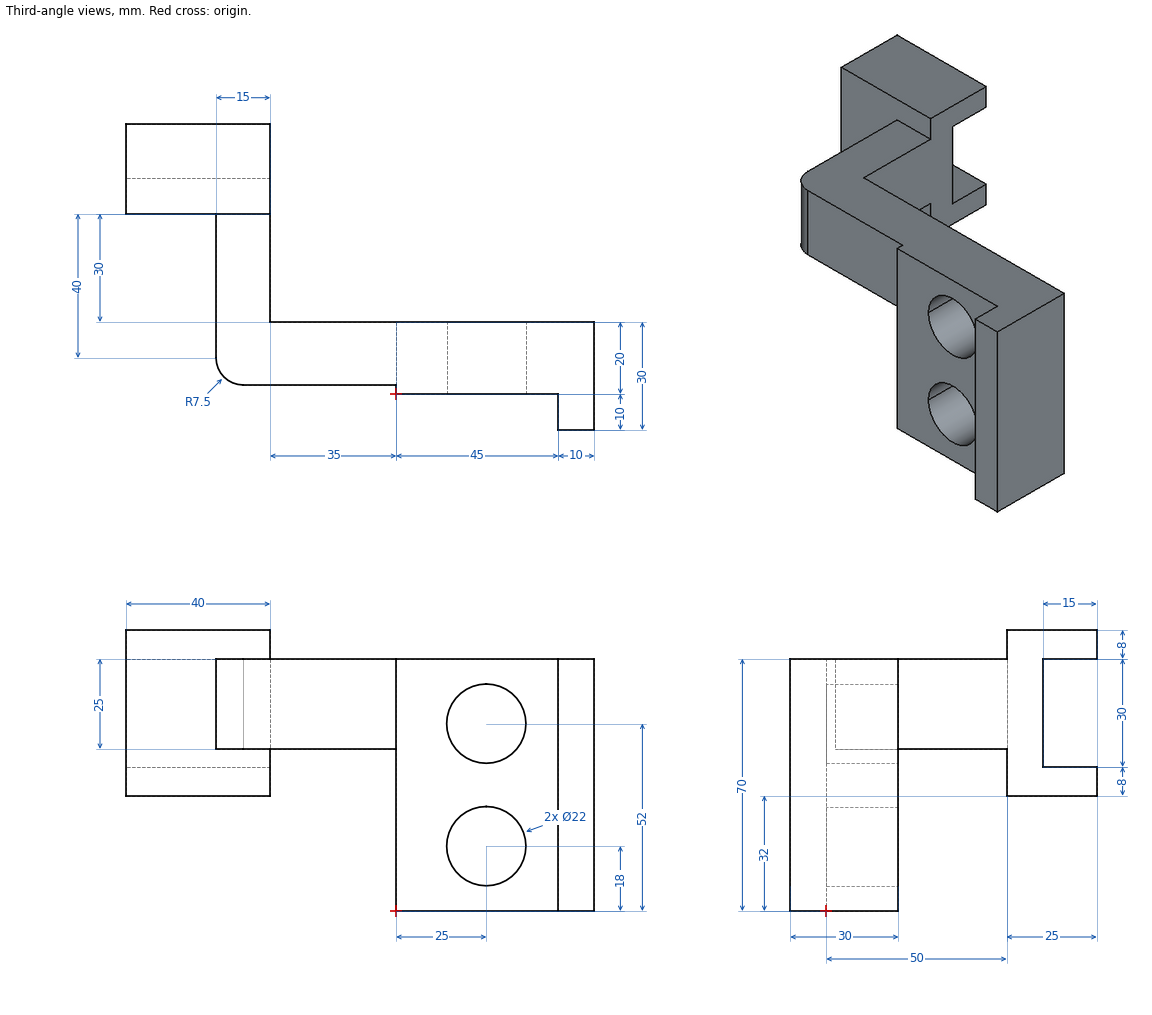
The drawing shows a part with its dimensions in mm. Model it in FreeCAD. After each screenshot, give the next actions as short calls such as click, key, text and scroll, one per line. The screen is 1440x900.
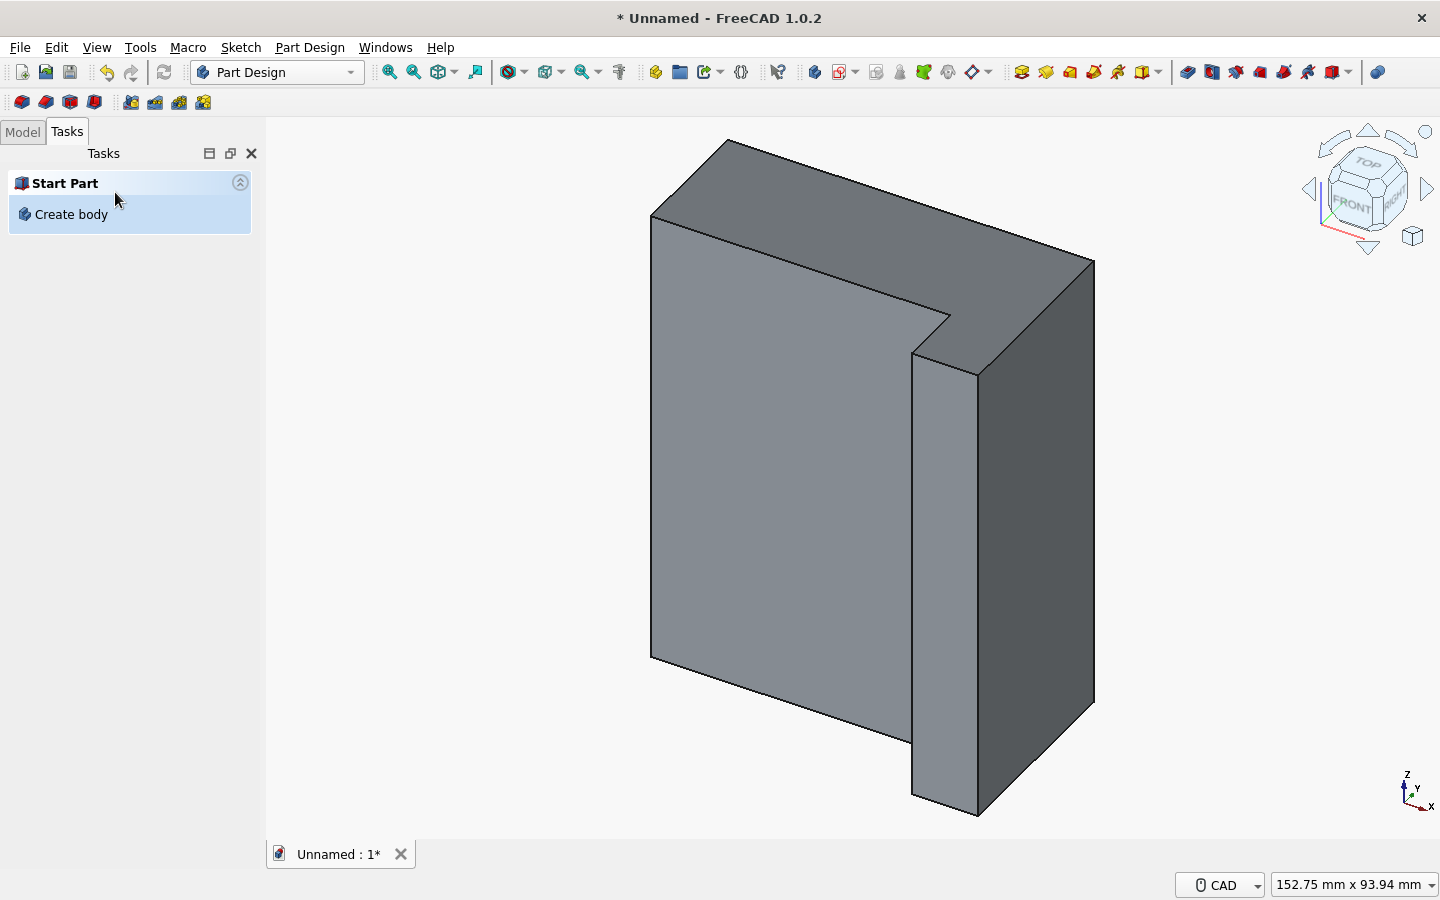
click(974, 275)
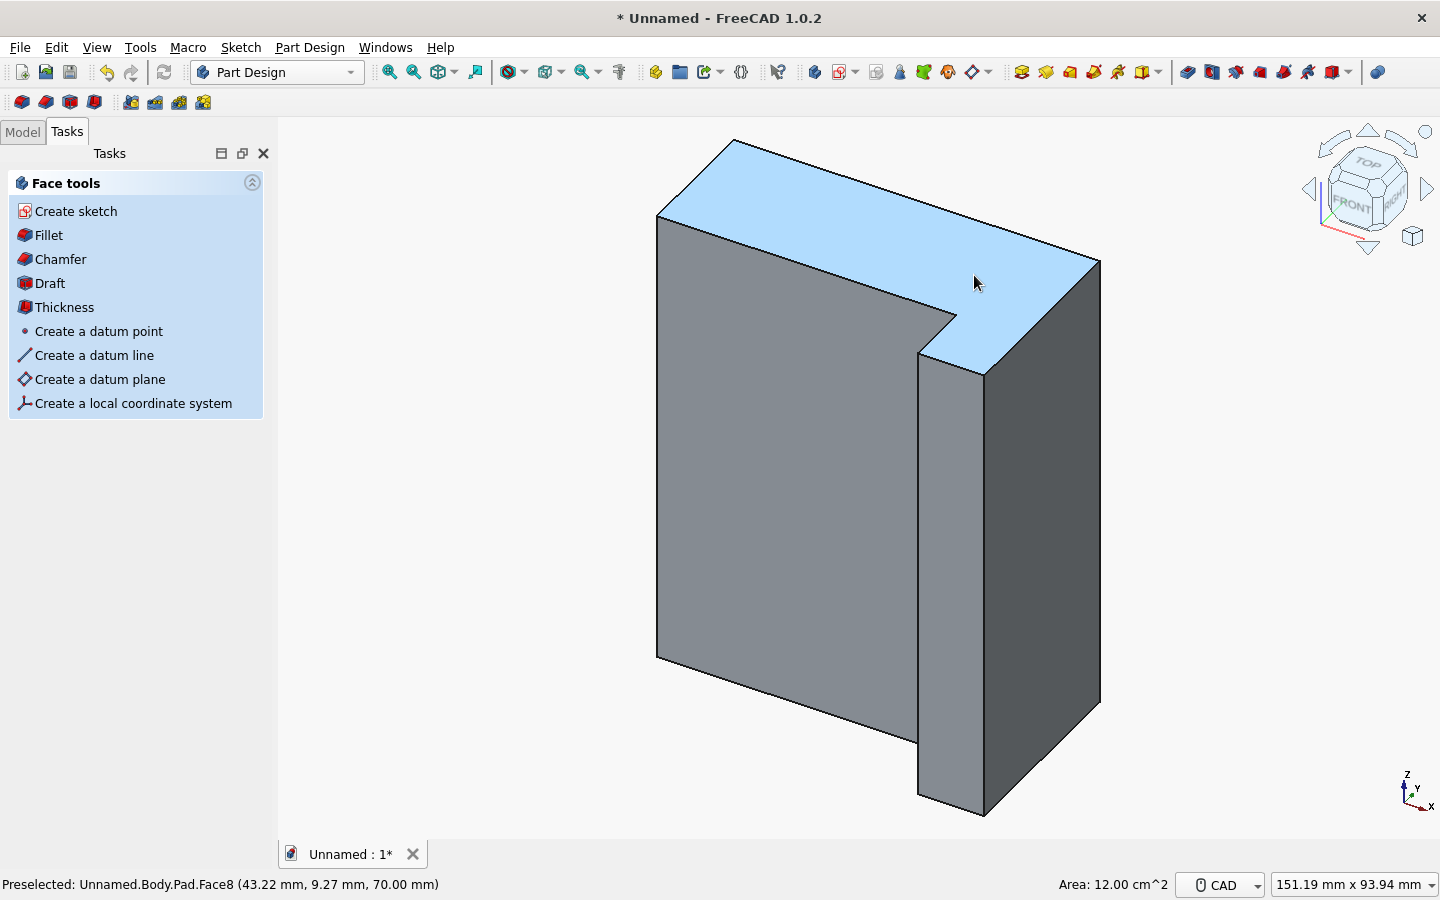
click(840, 72)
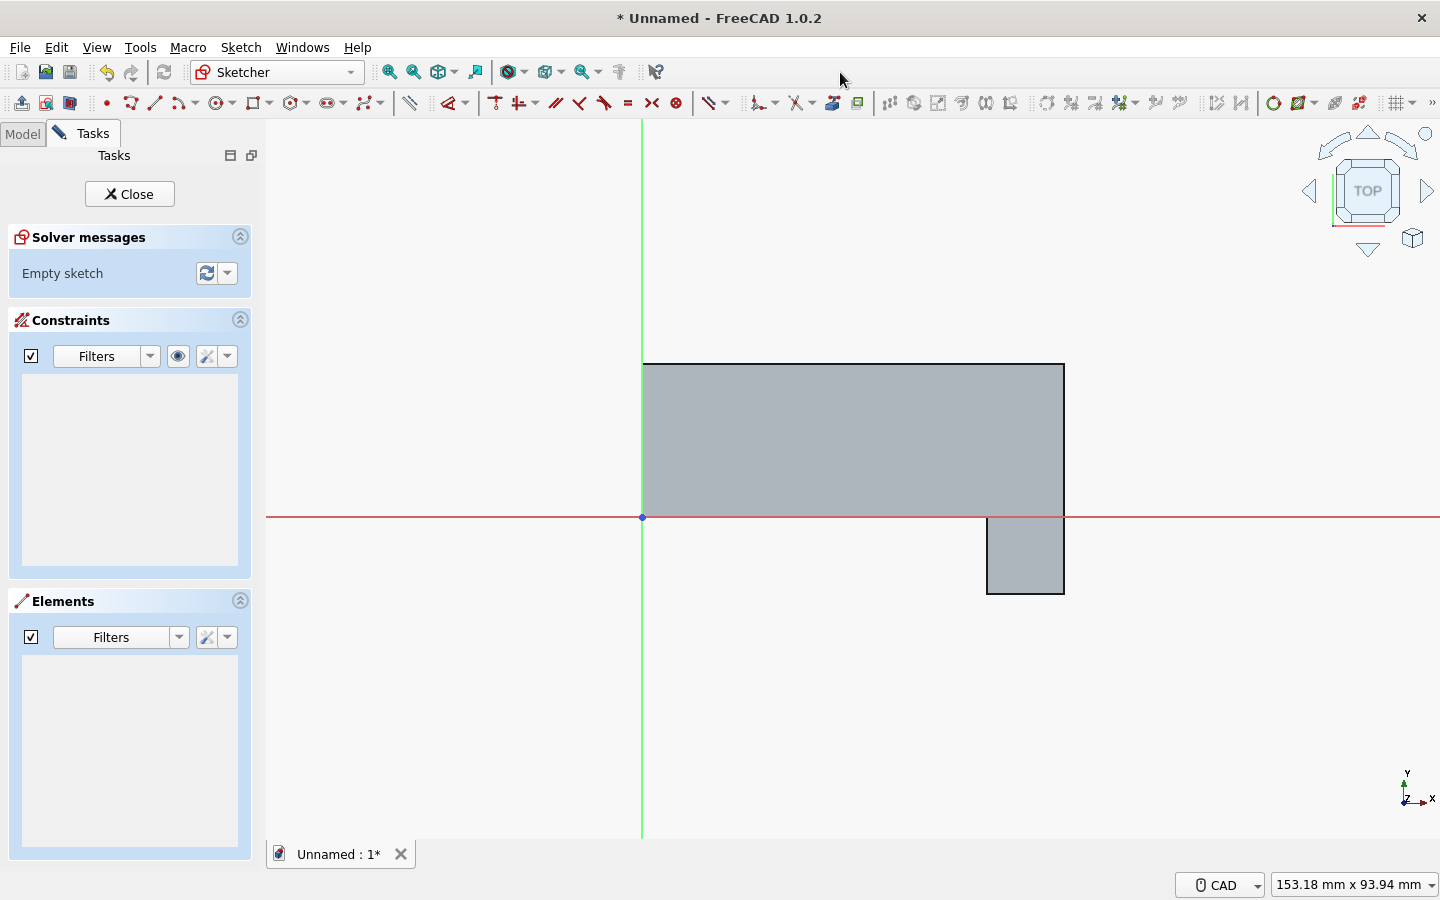
scroll(1275, 811, down, 1)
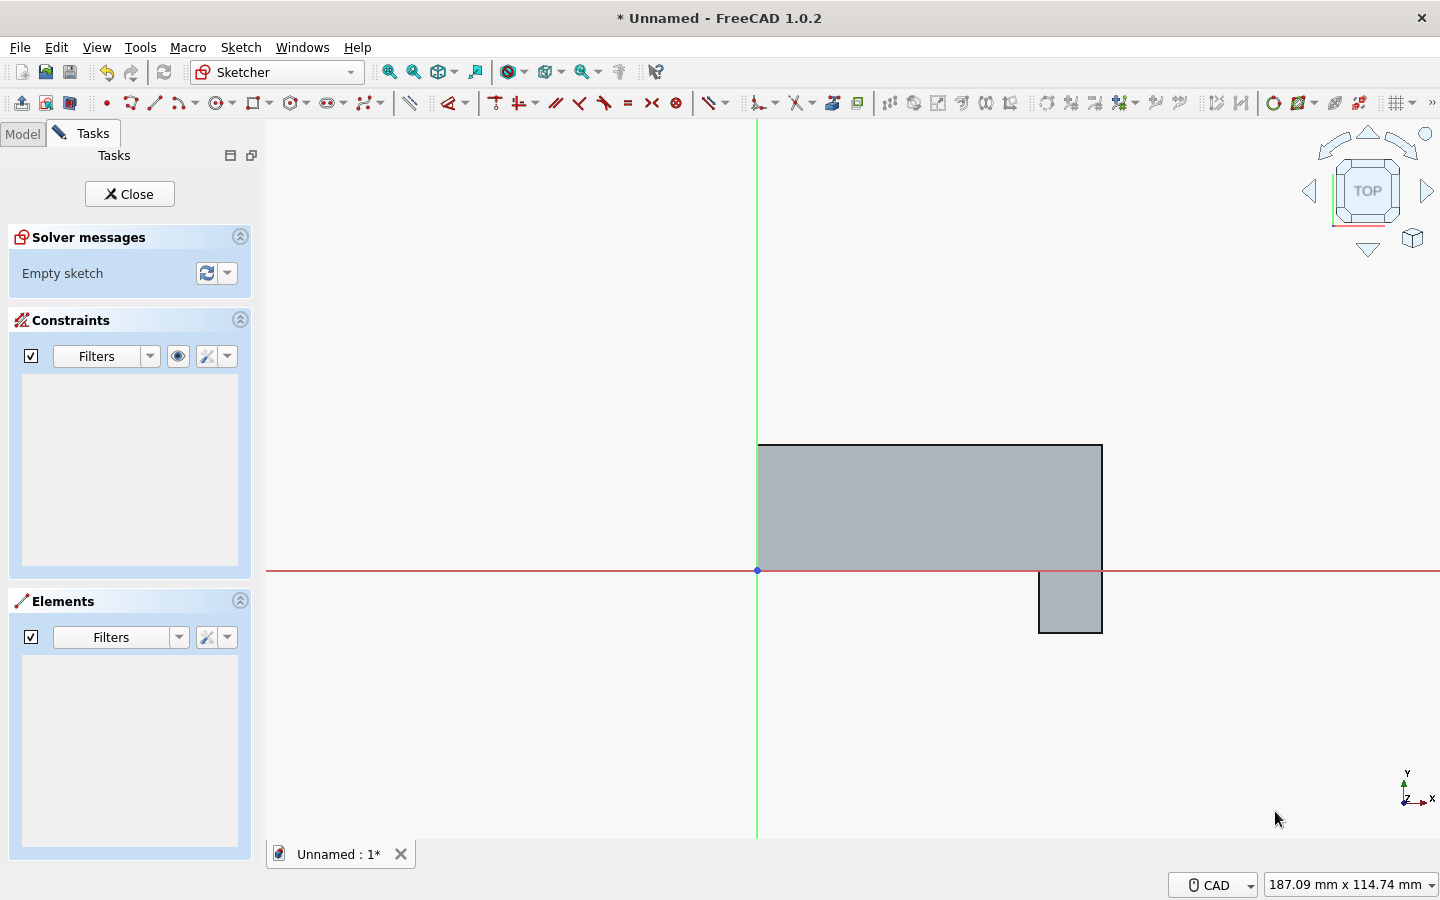
scroll(294, 281, up, 2)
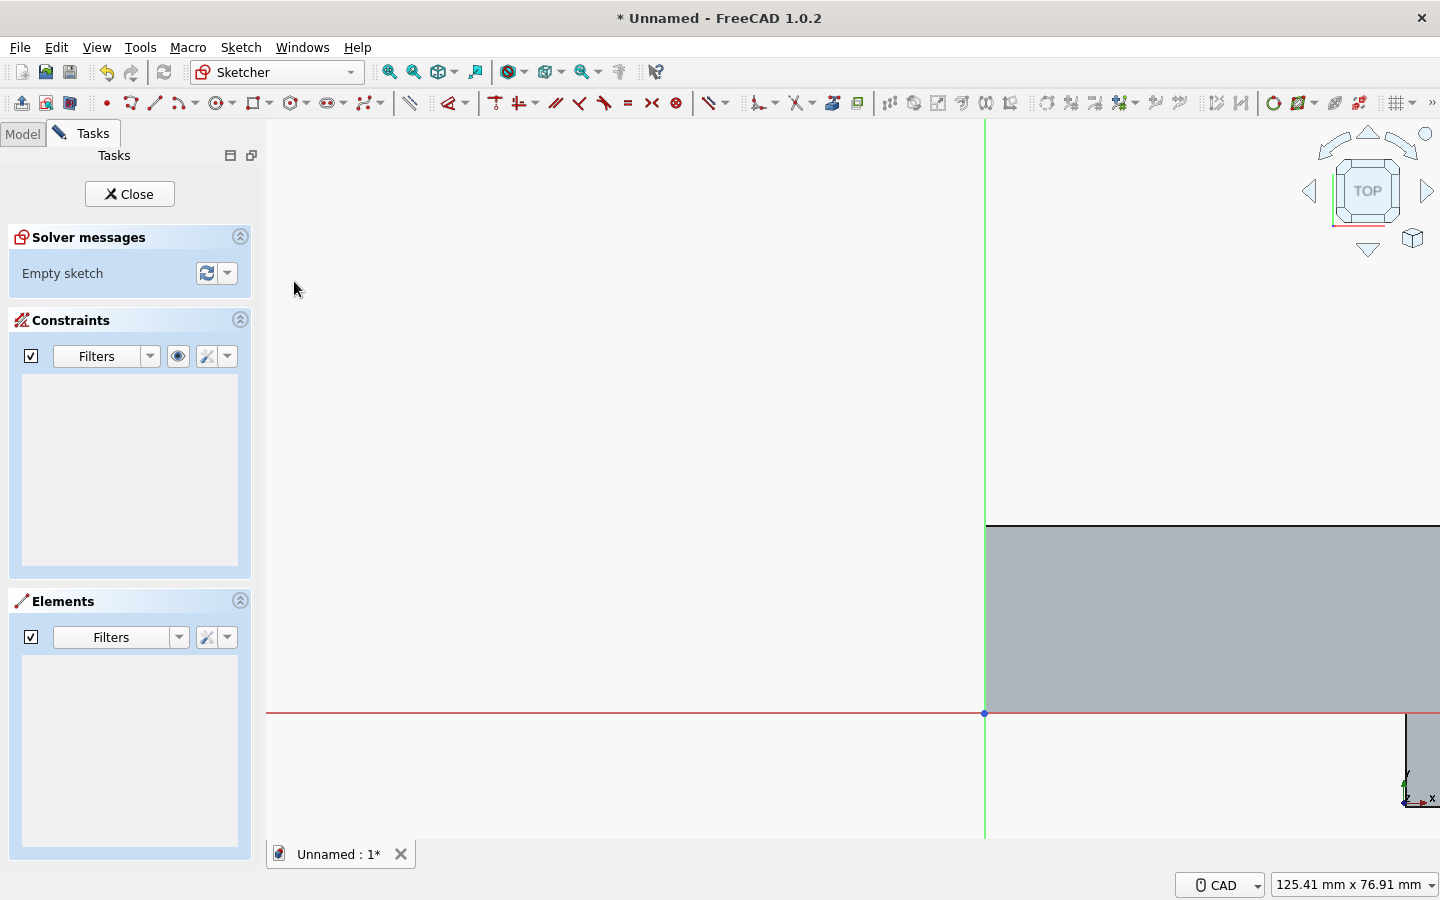
click(132, 104)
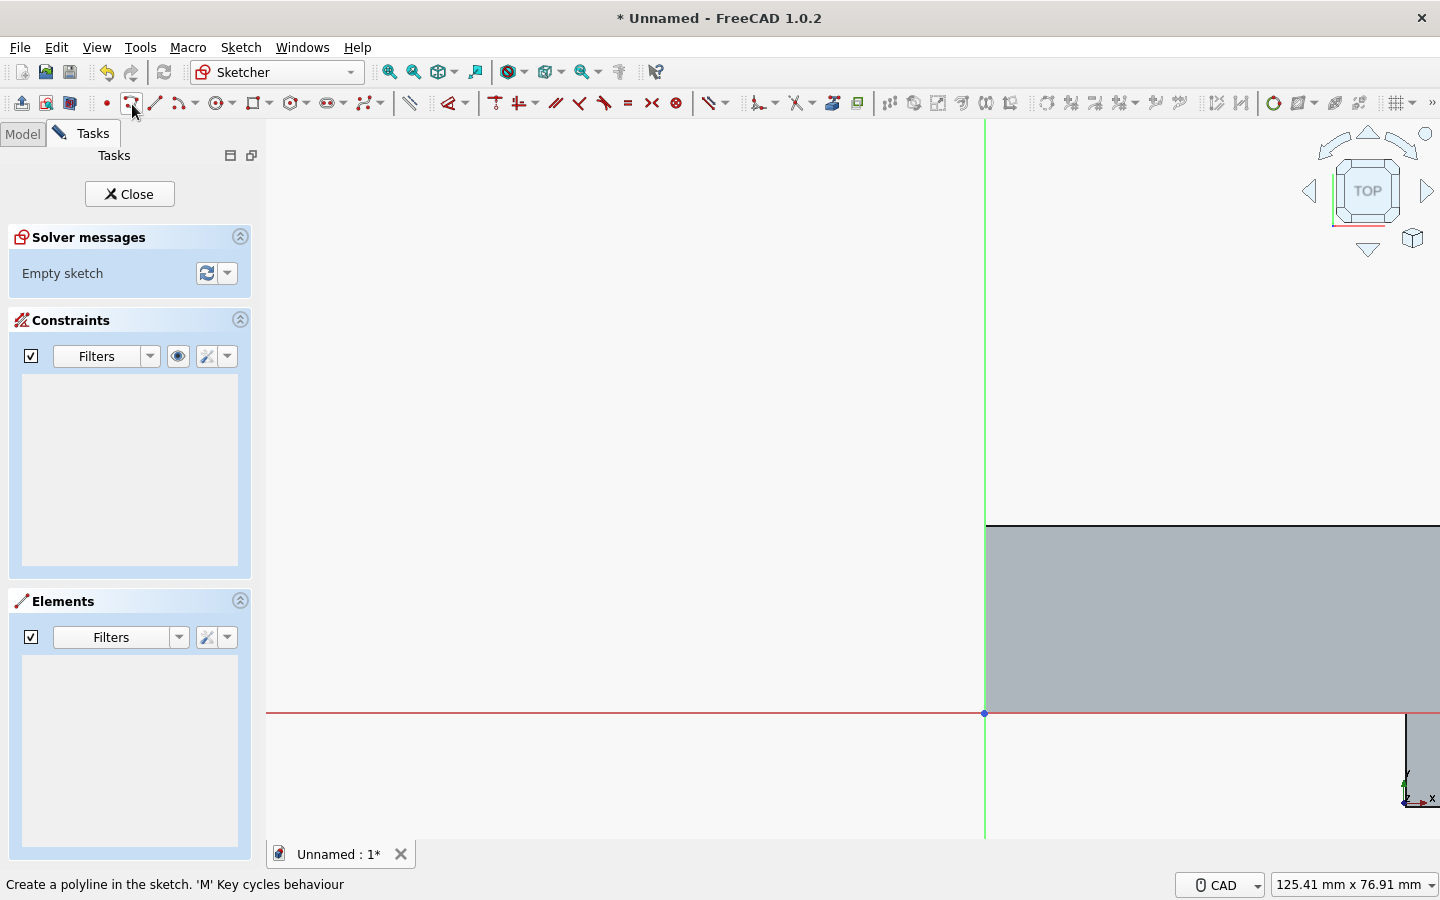
click(587, 690)
click(985, 690)
click(976, 526)
click(657, 526)
click(657, 245)
click(517, 245)
click(517, 620)
right_click(517, 620)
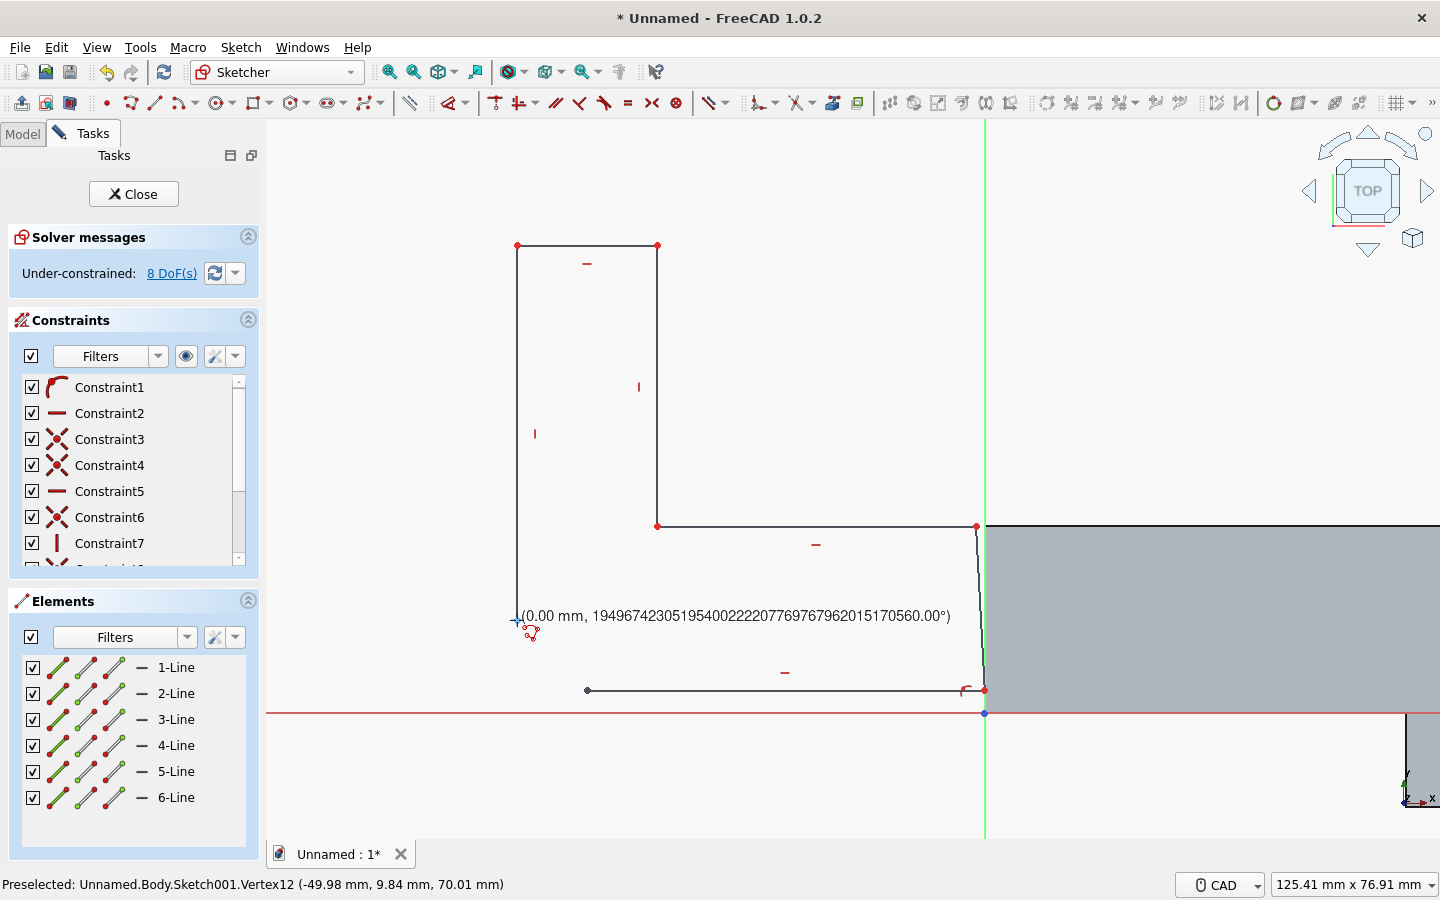
click(198, 104)